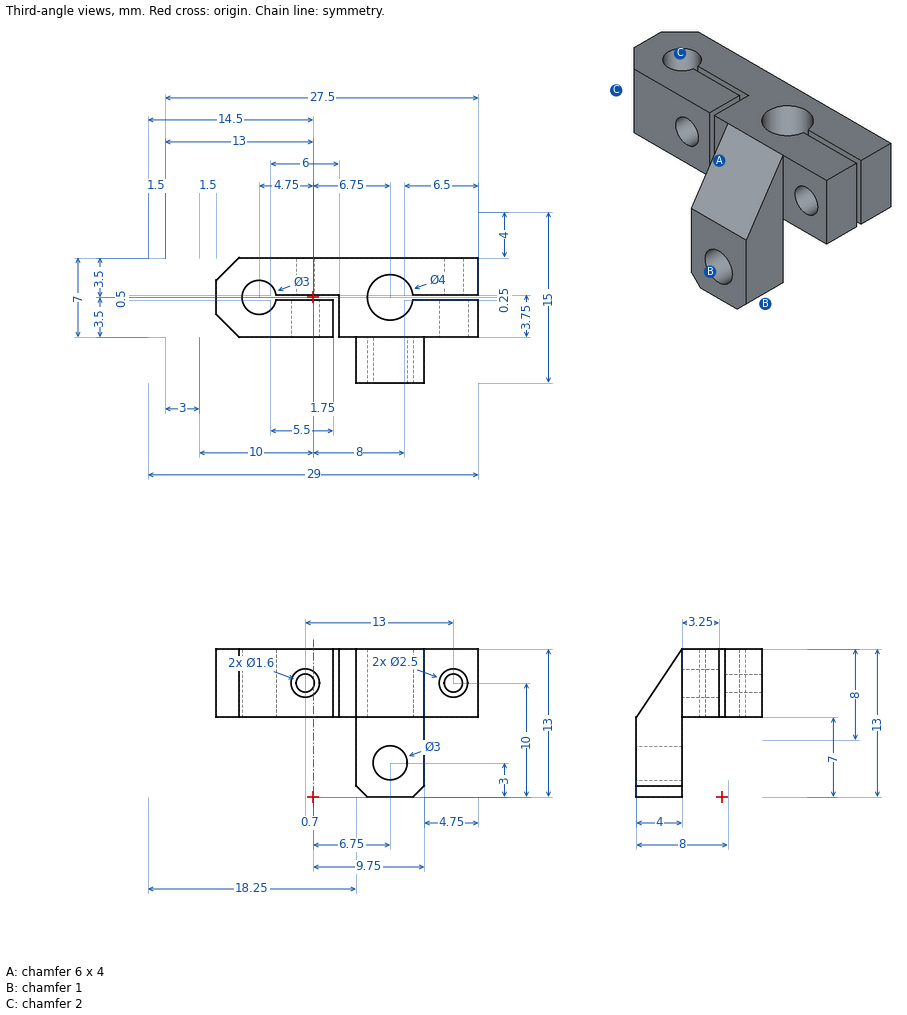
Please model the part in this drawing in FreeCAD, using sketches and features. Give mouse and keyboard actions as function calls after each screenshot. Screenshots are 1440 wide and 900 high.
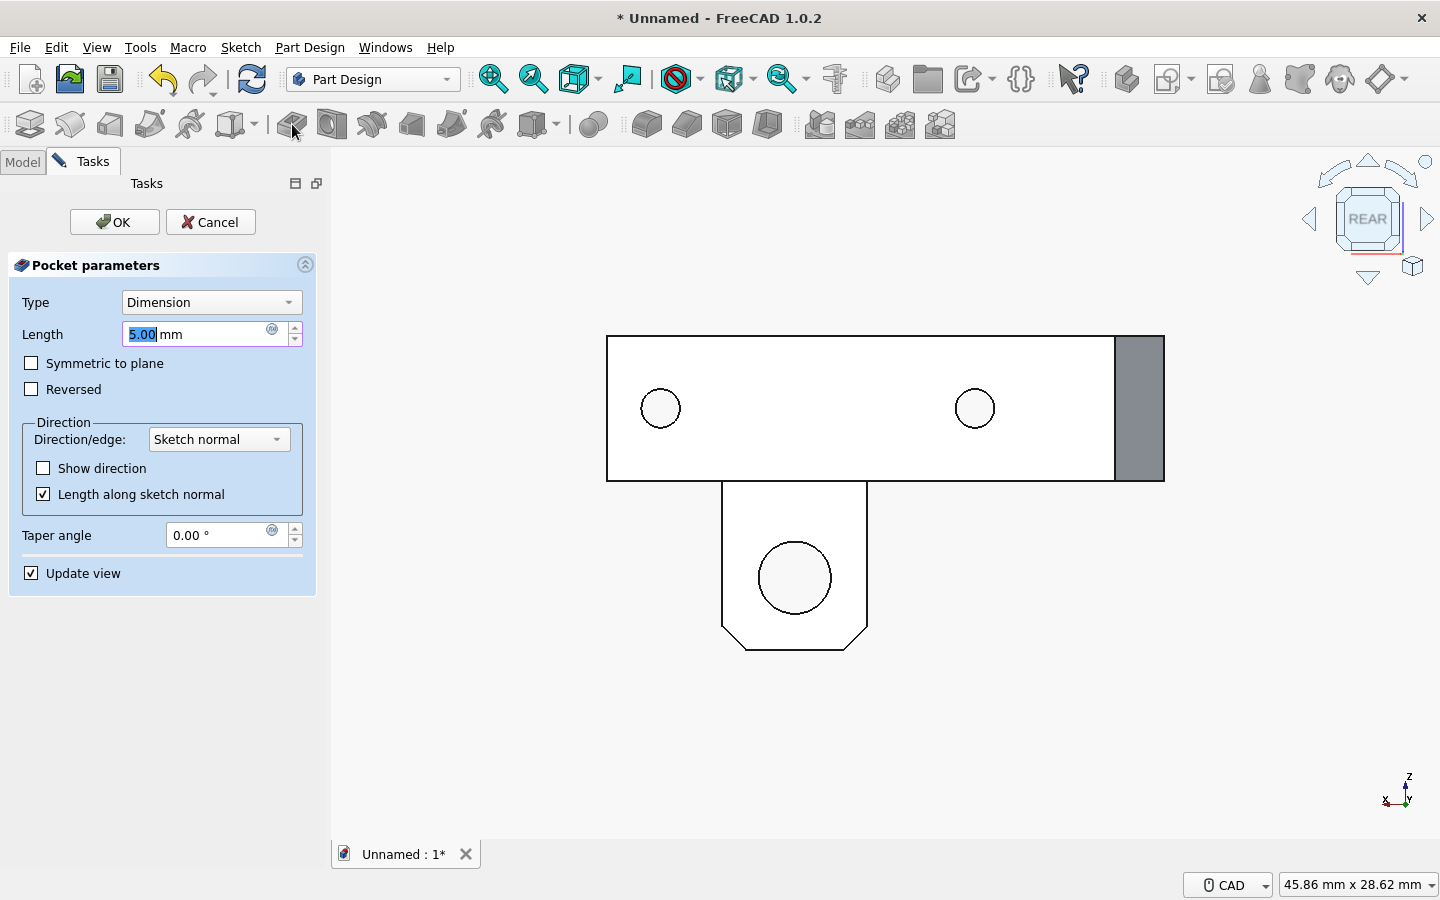
click(212, 302)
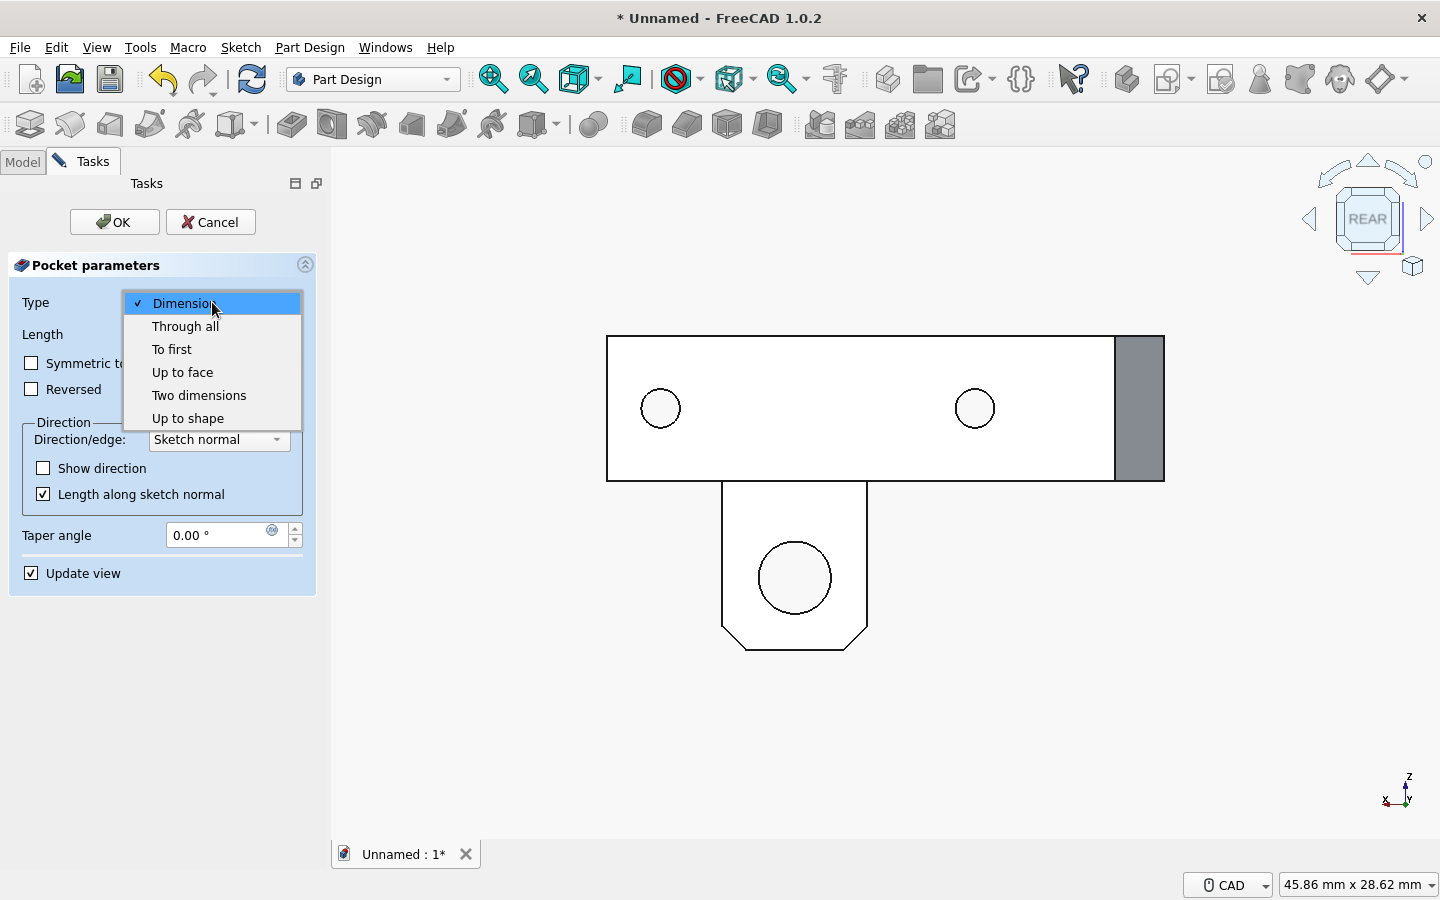
click(212, 326)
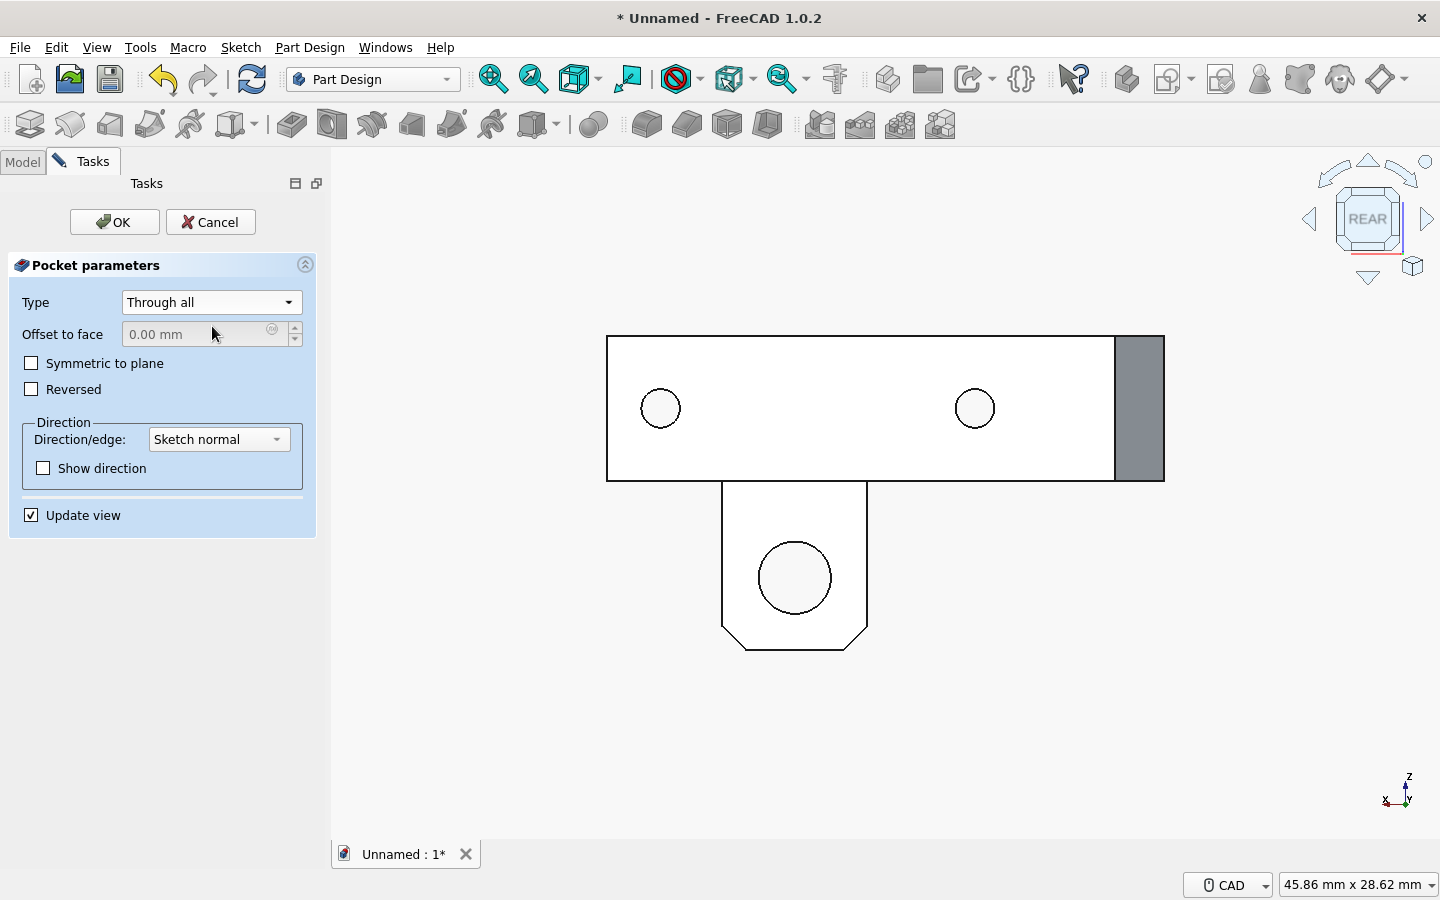
click(115, 222)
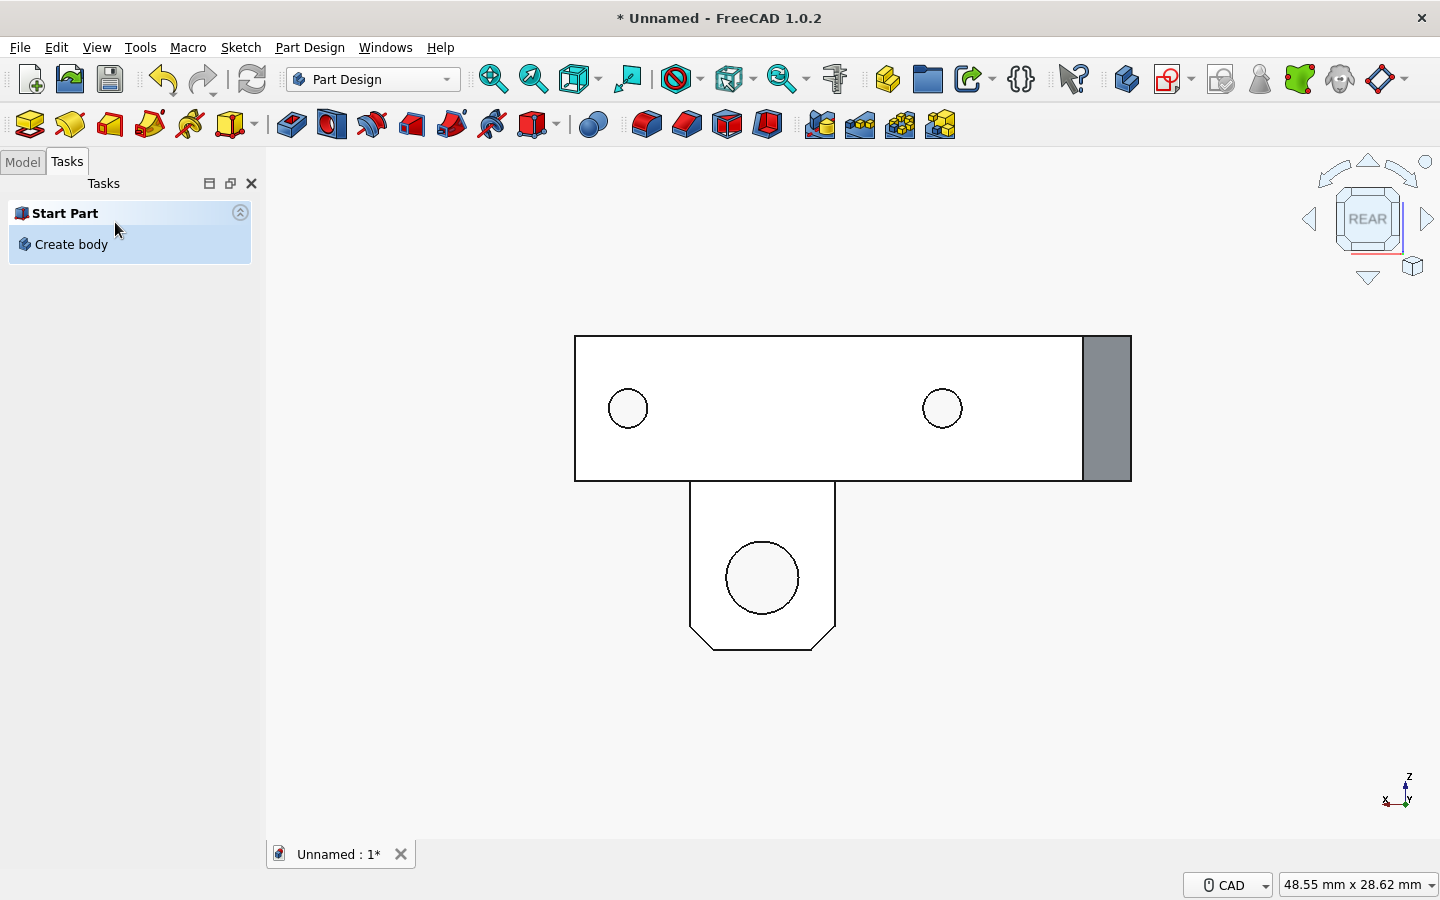
key(0)